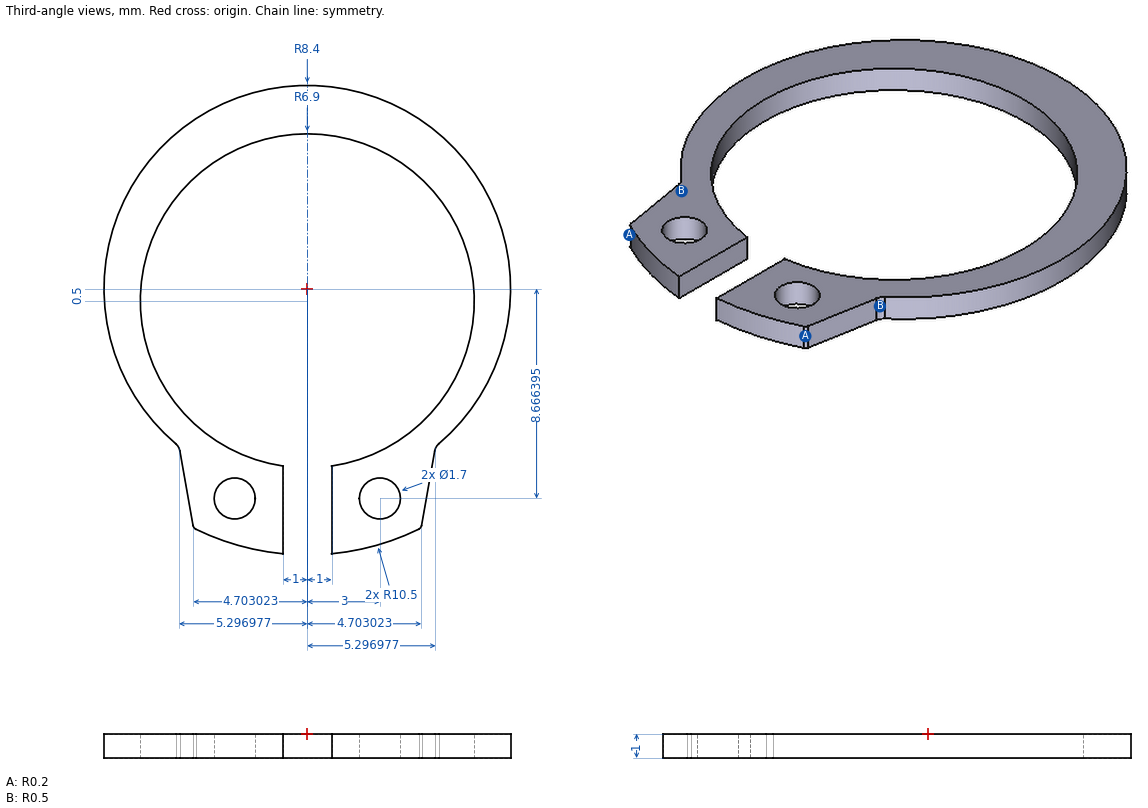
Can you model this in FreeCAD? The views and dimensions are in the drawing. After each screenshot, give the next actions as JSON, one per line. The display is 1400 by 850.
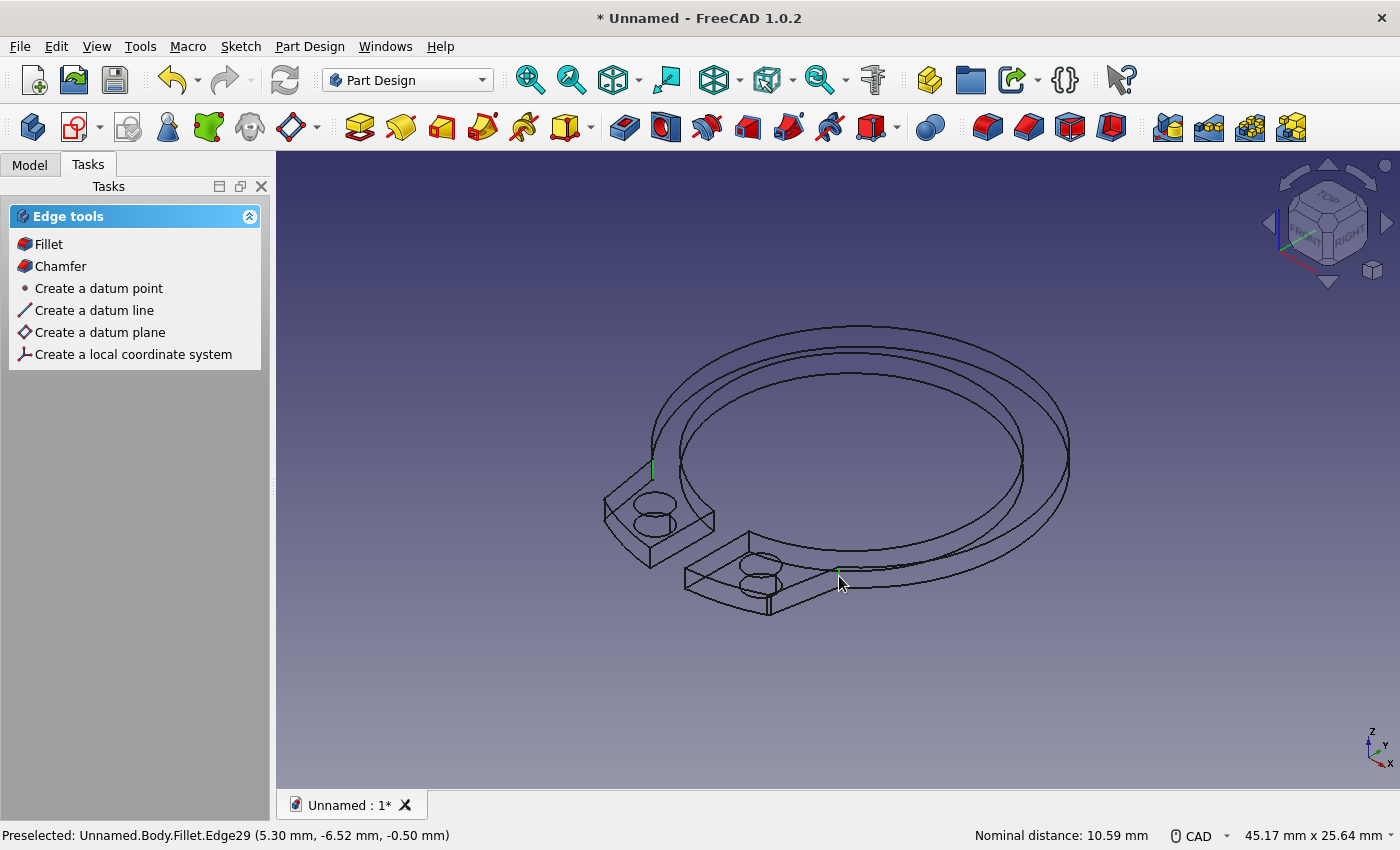
{"action": "key", "text": "v 1"}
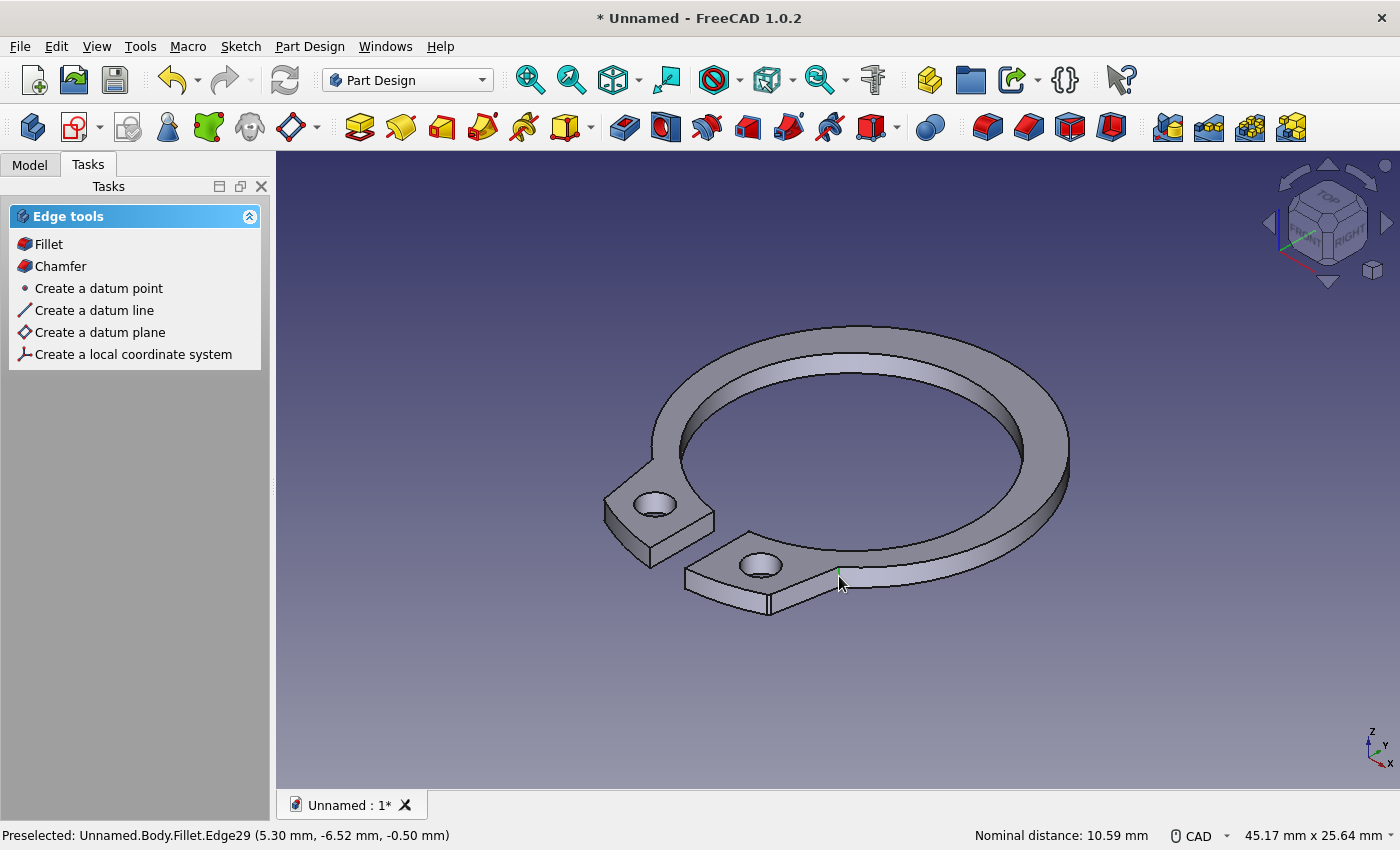
{"action": "left_click", "coordinate": [988, 128]}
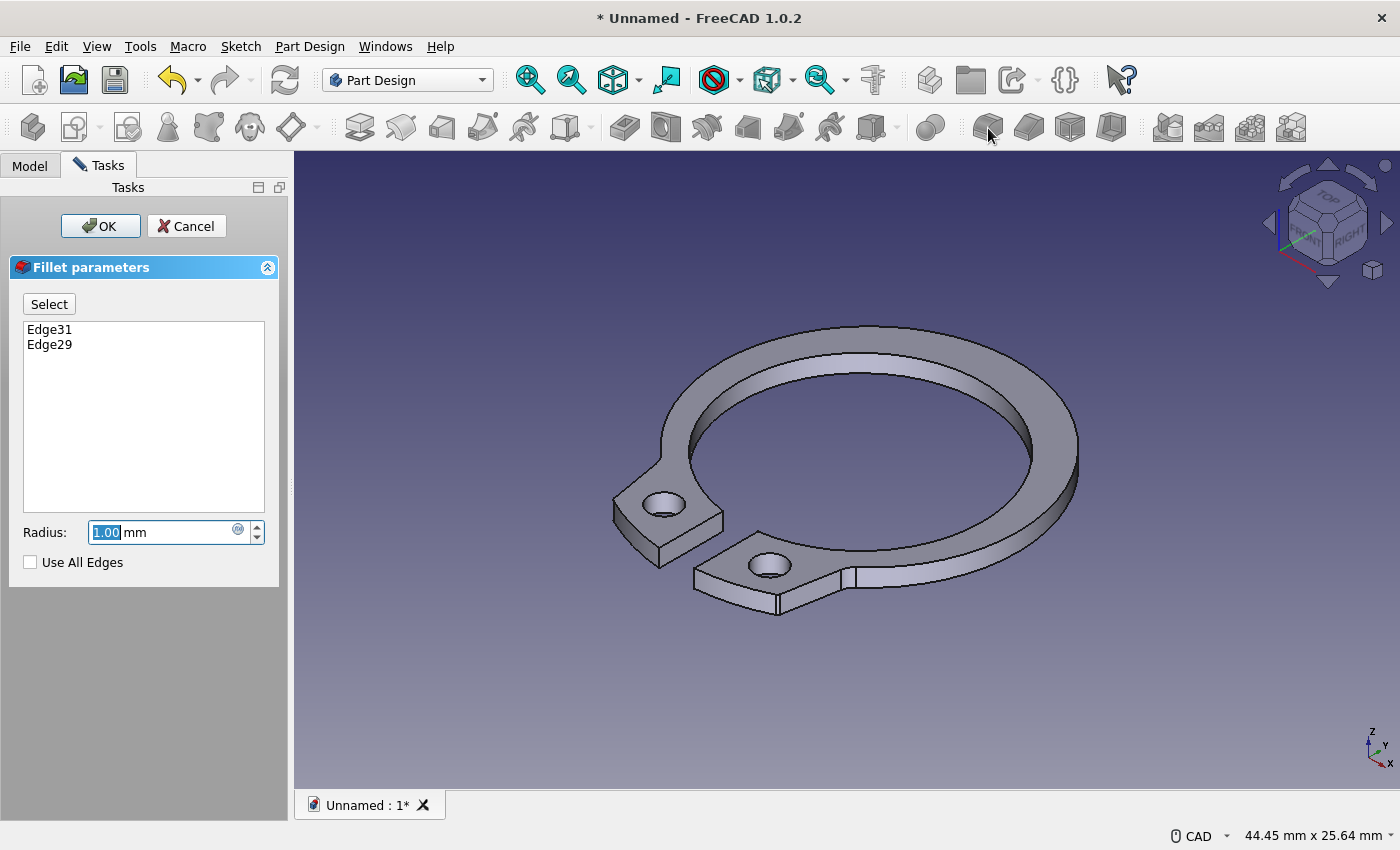
{"action": "type", "text": "0.5"}
{"action": "key", "text": "Tab"}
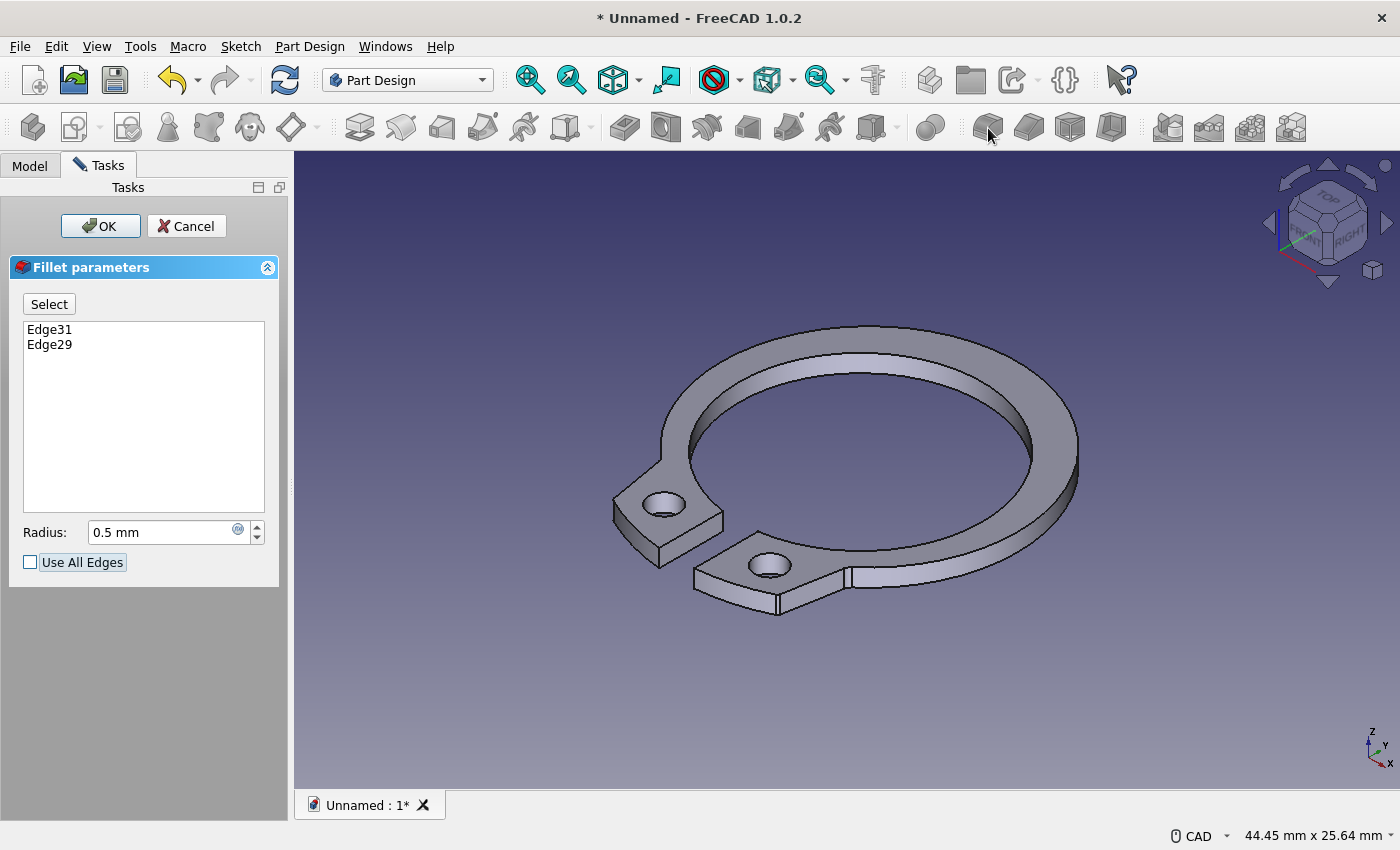
{"action": "left_click", "coordinate": [101, 226]}